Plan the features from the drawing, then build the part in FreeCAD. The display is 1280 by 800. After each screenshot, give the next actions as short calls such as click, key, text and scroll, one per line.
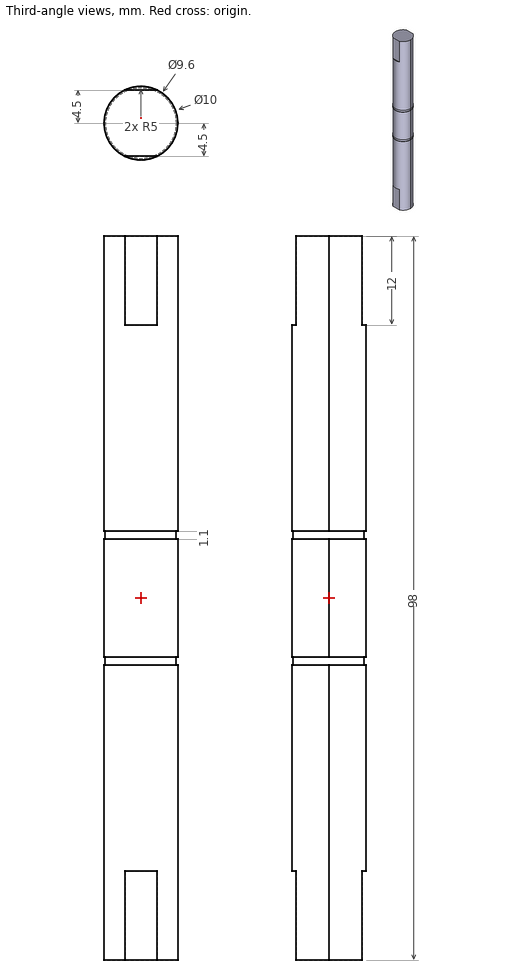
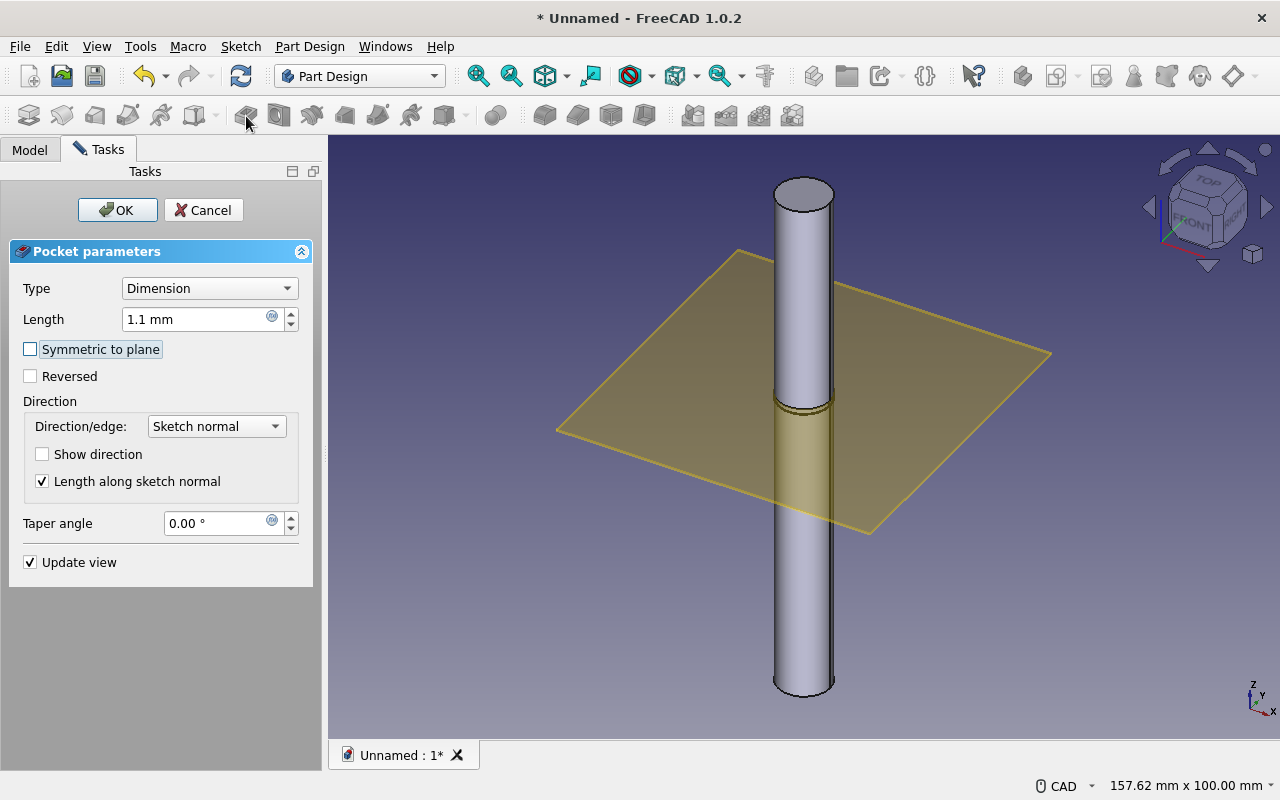
click(118, 210)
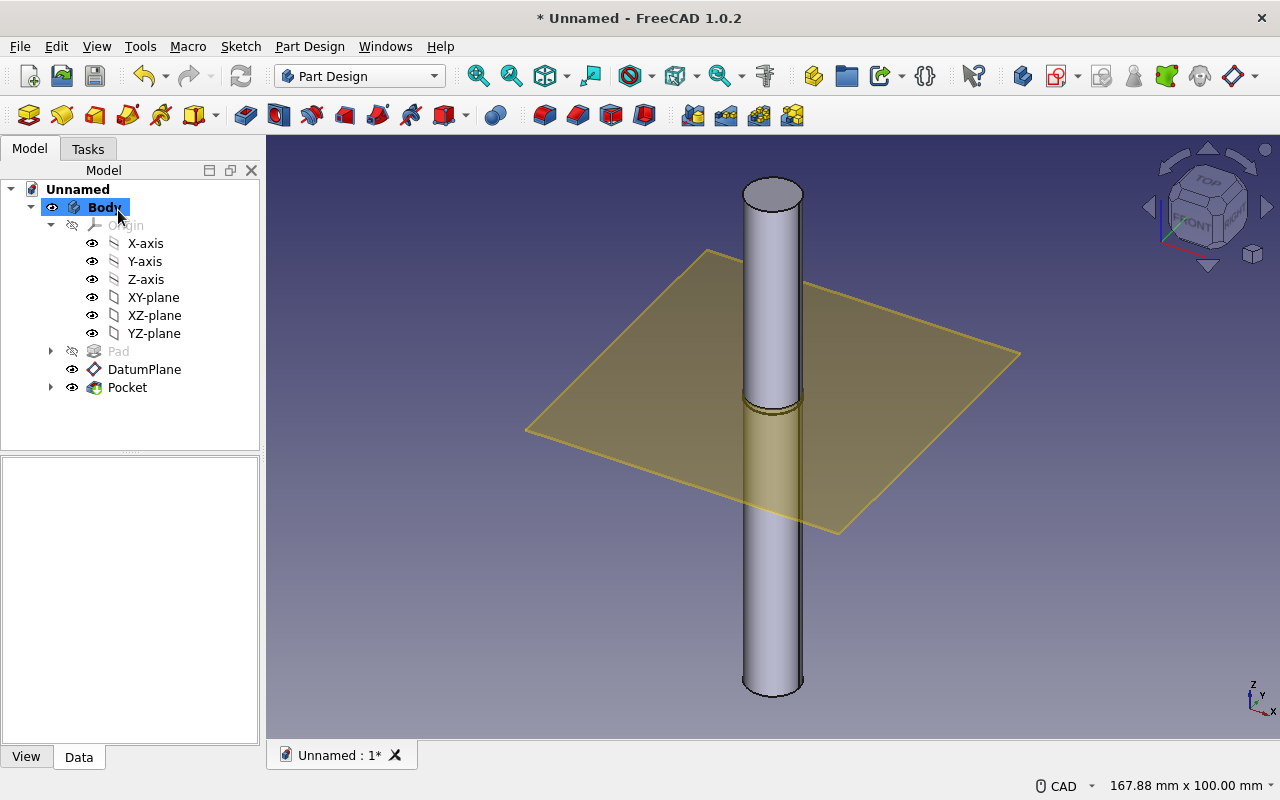
click(117, 369)
key(space)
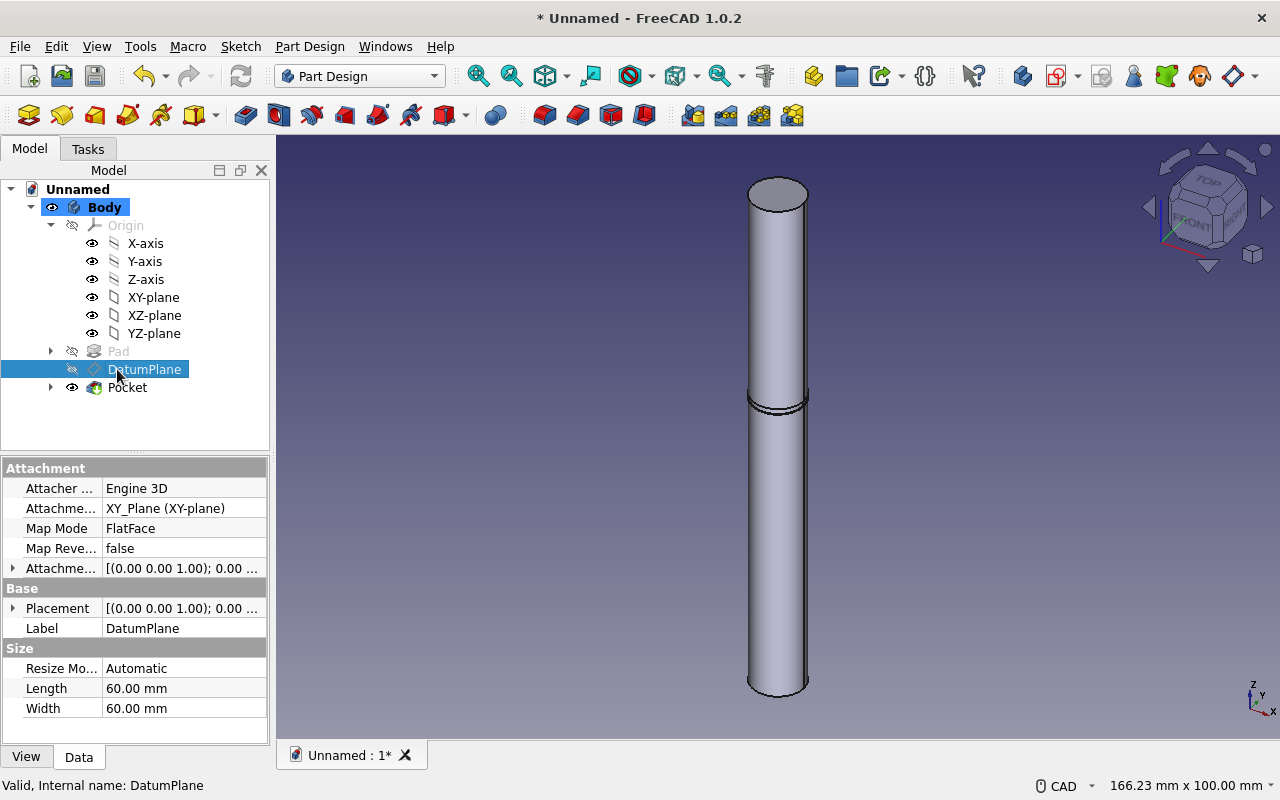
click(117, 387)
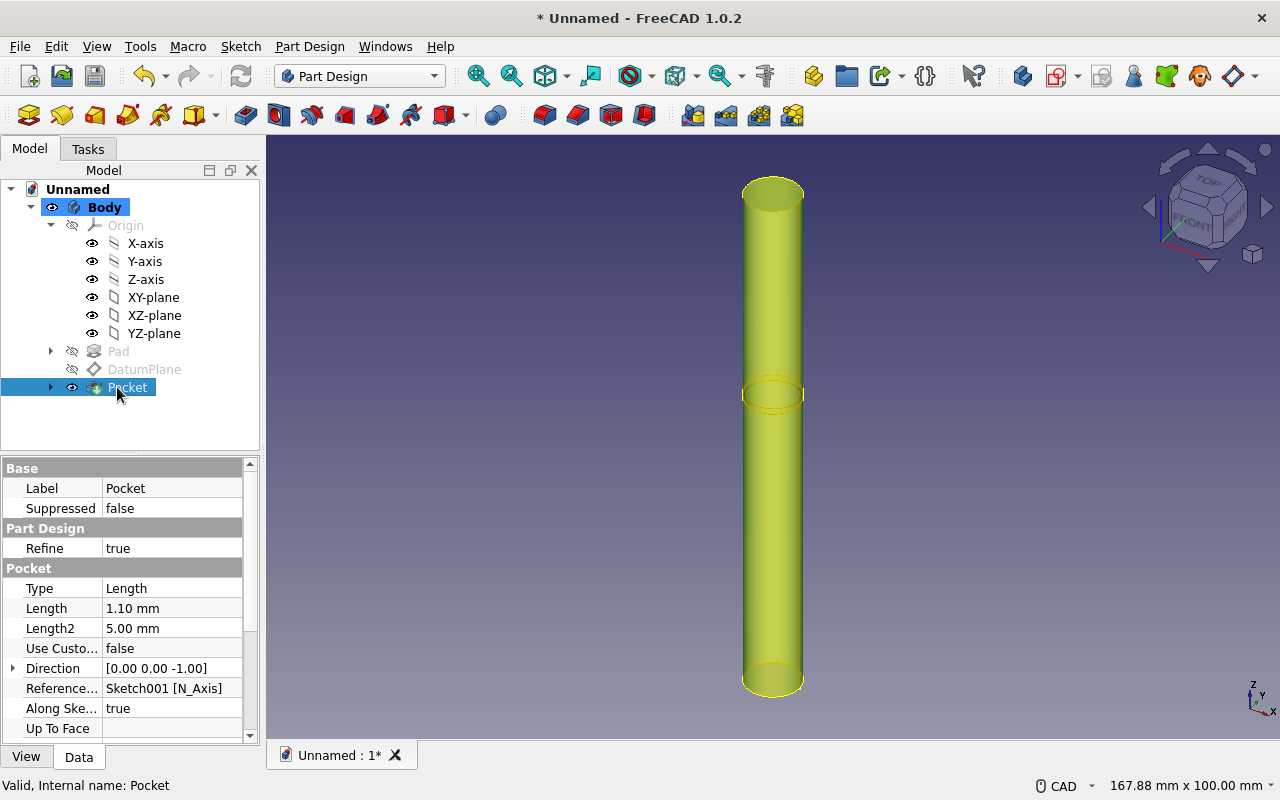
click(693, 116)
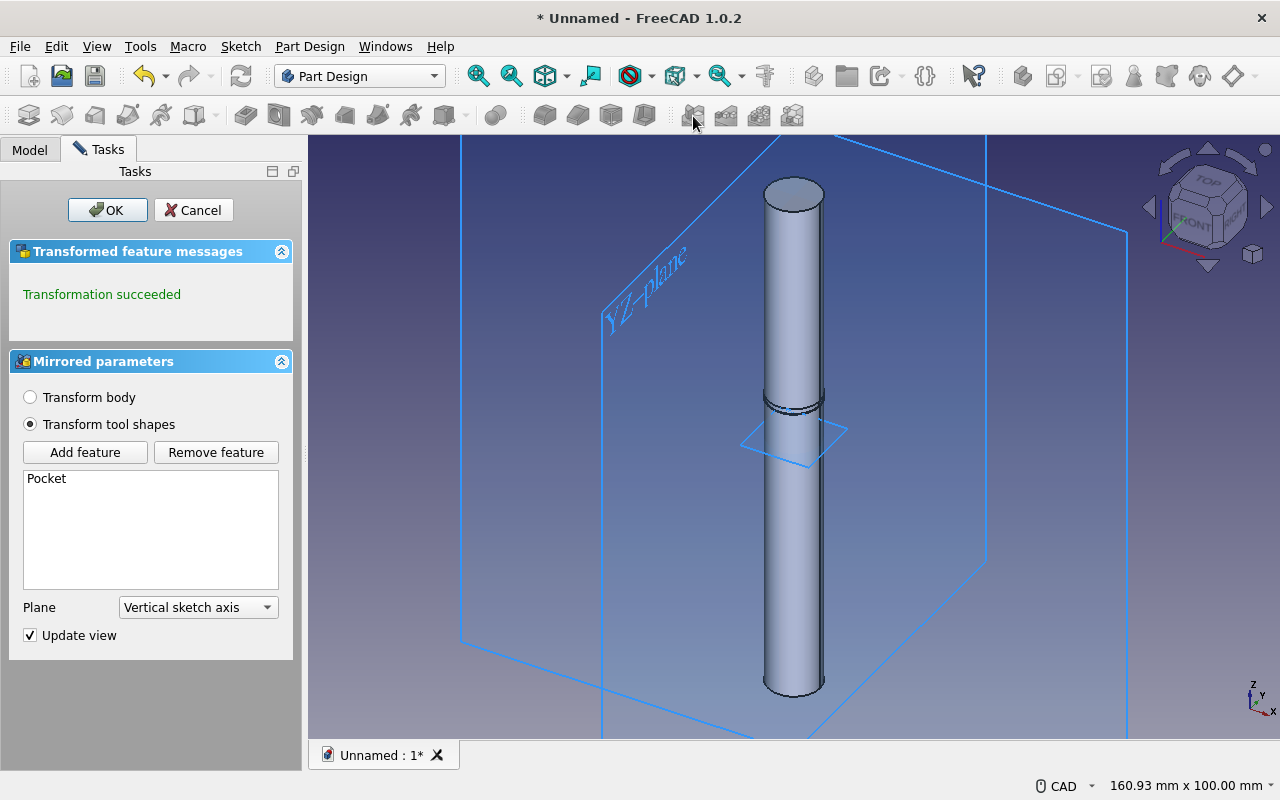
click(199, 608)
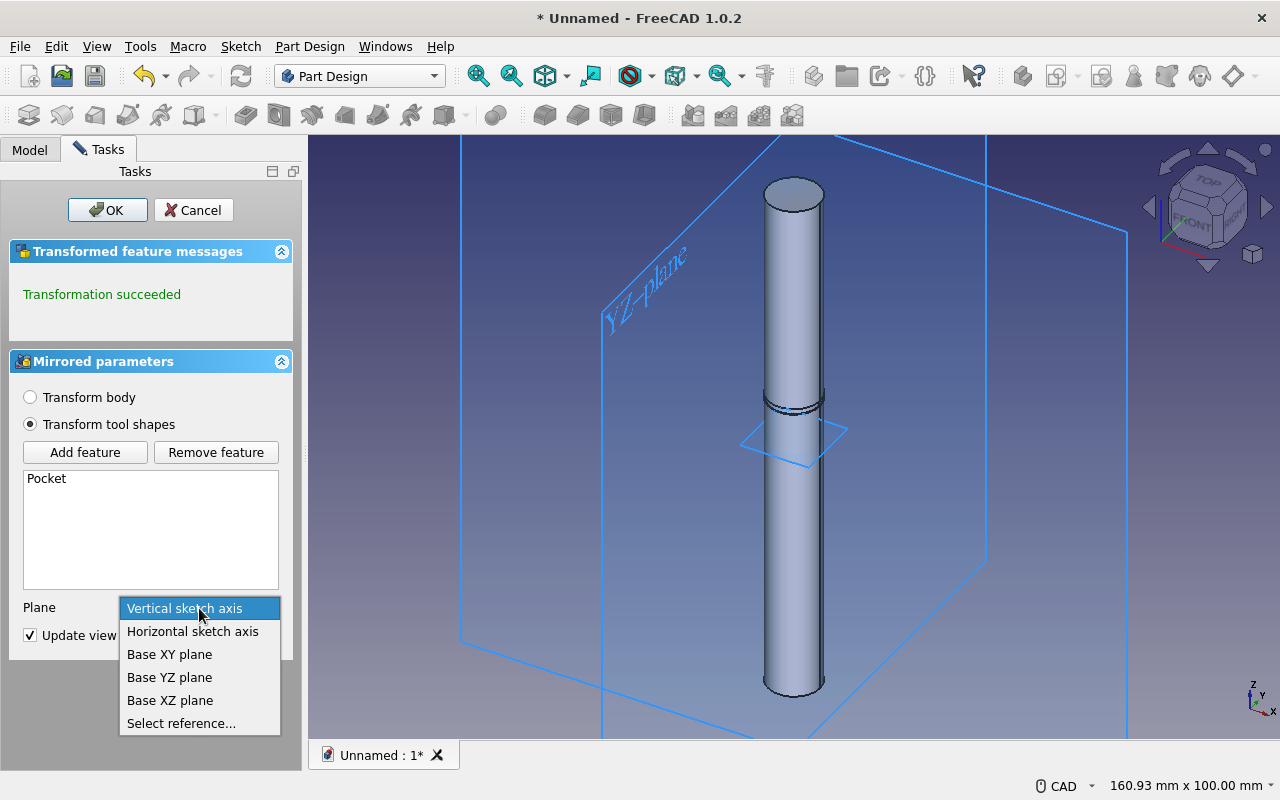
click(198, 654)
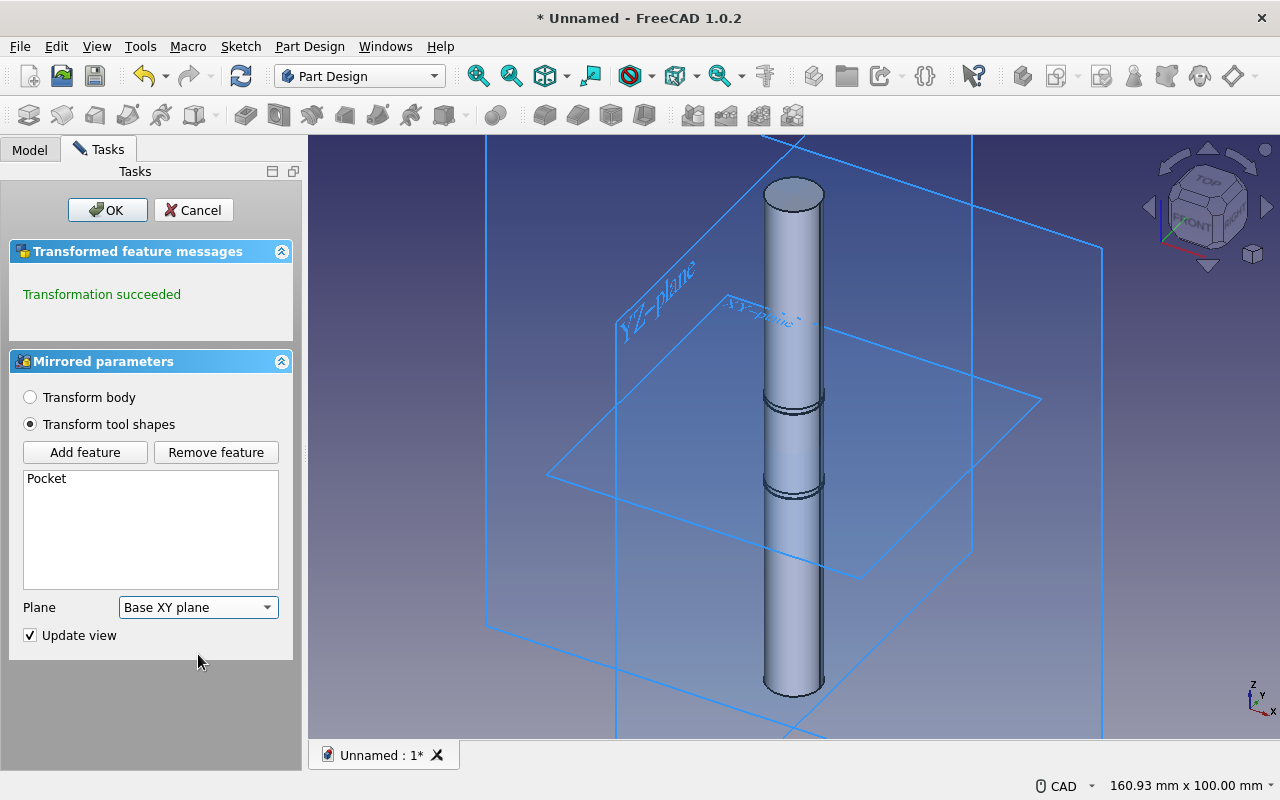
click(108, 210)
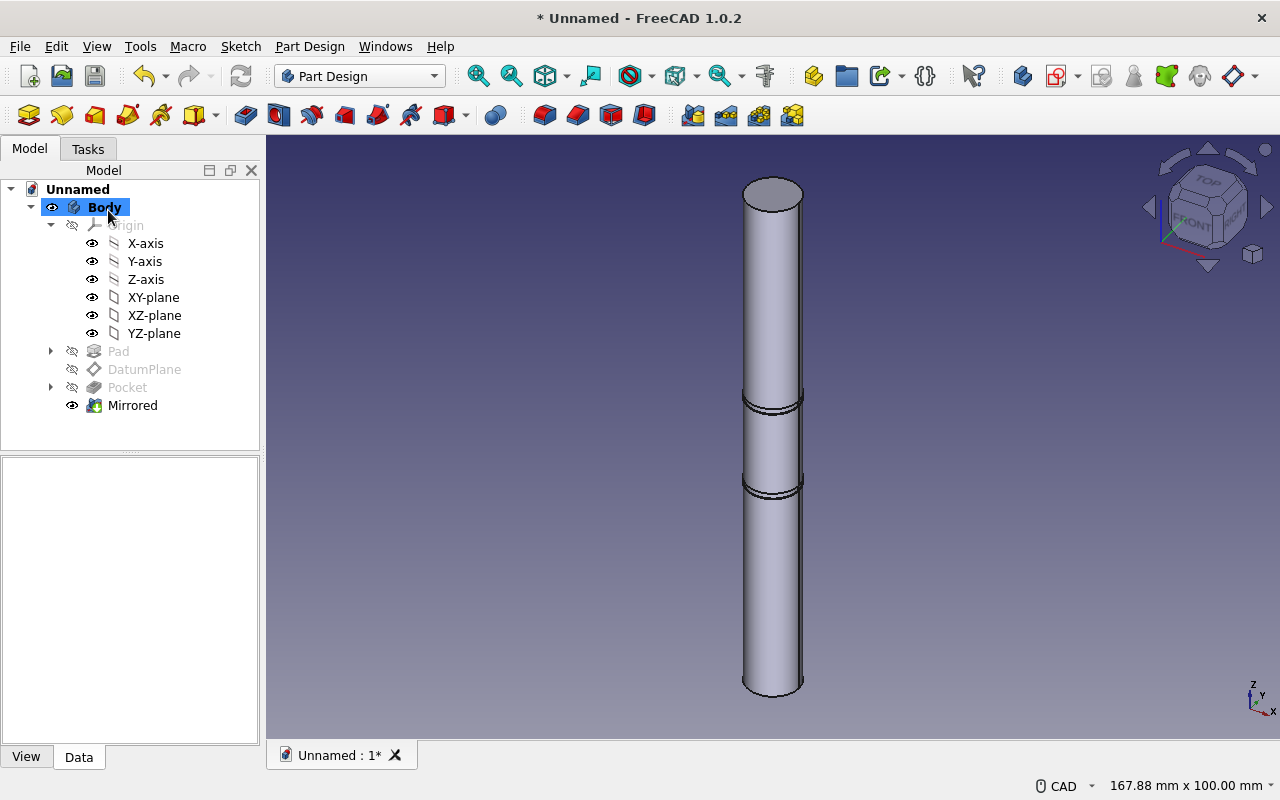
click(773, 194)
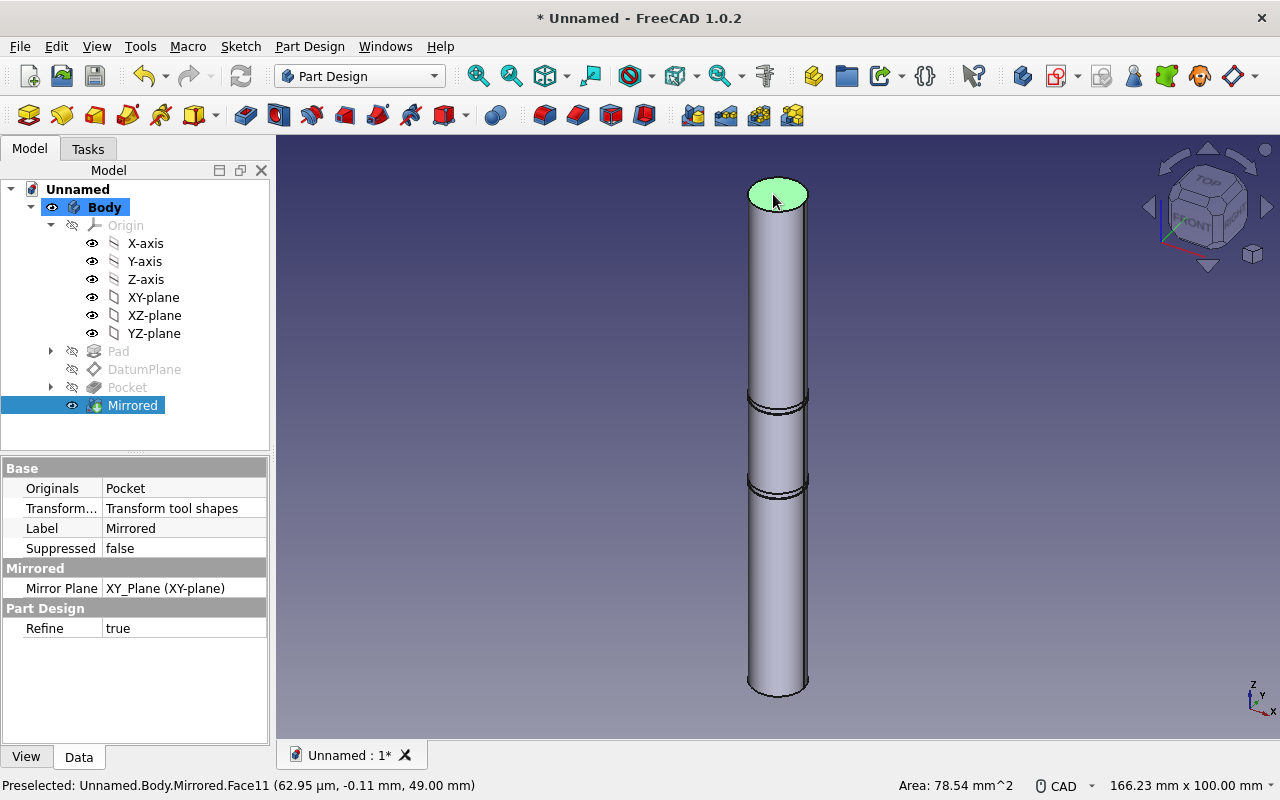
click(1056, 76)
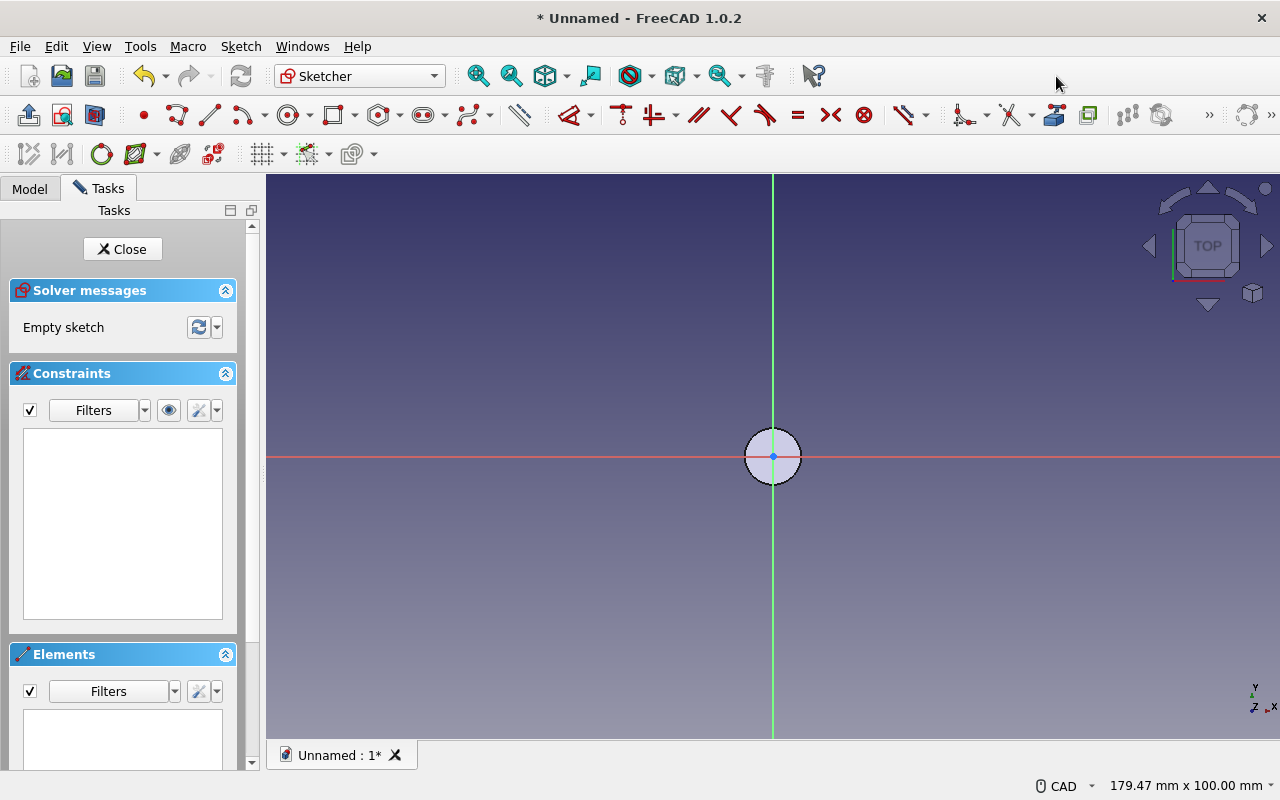
scroll(787, 456, up, 9)